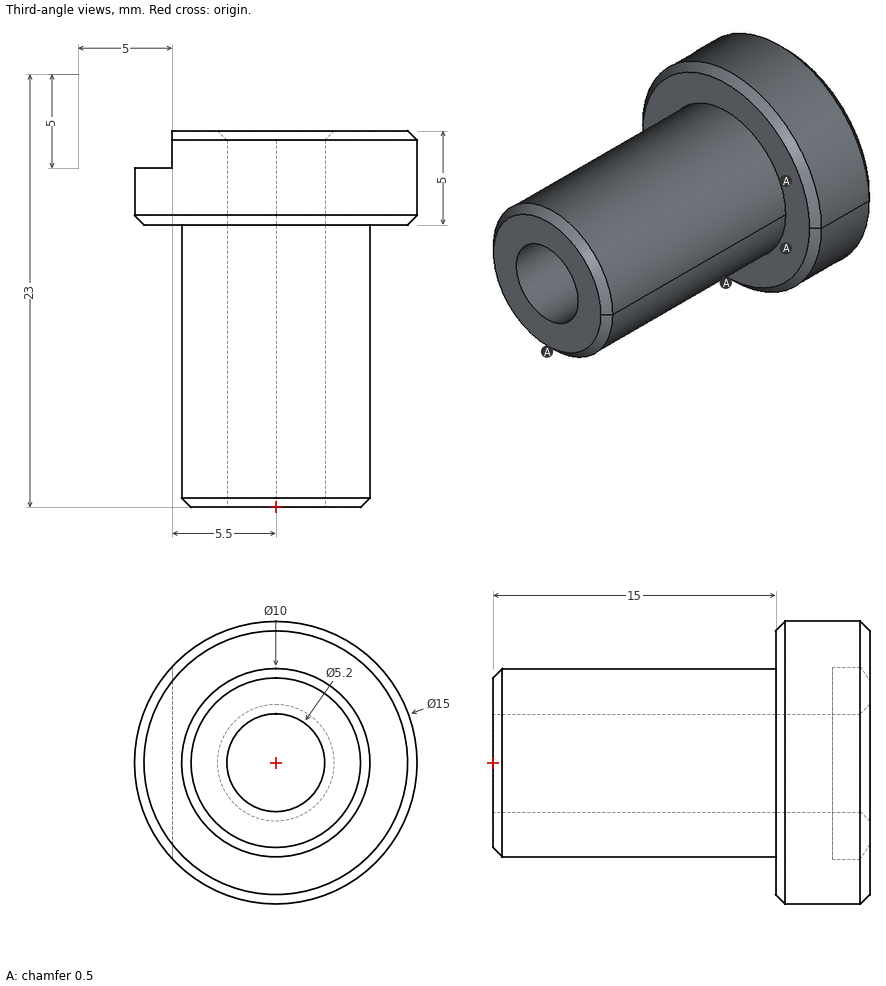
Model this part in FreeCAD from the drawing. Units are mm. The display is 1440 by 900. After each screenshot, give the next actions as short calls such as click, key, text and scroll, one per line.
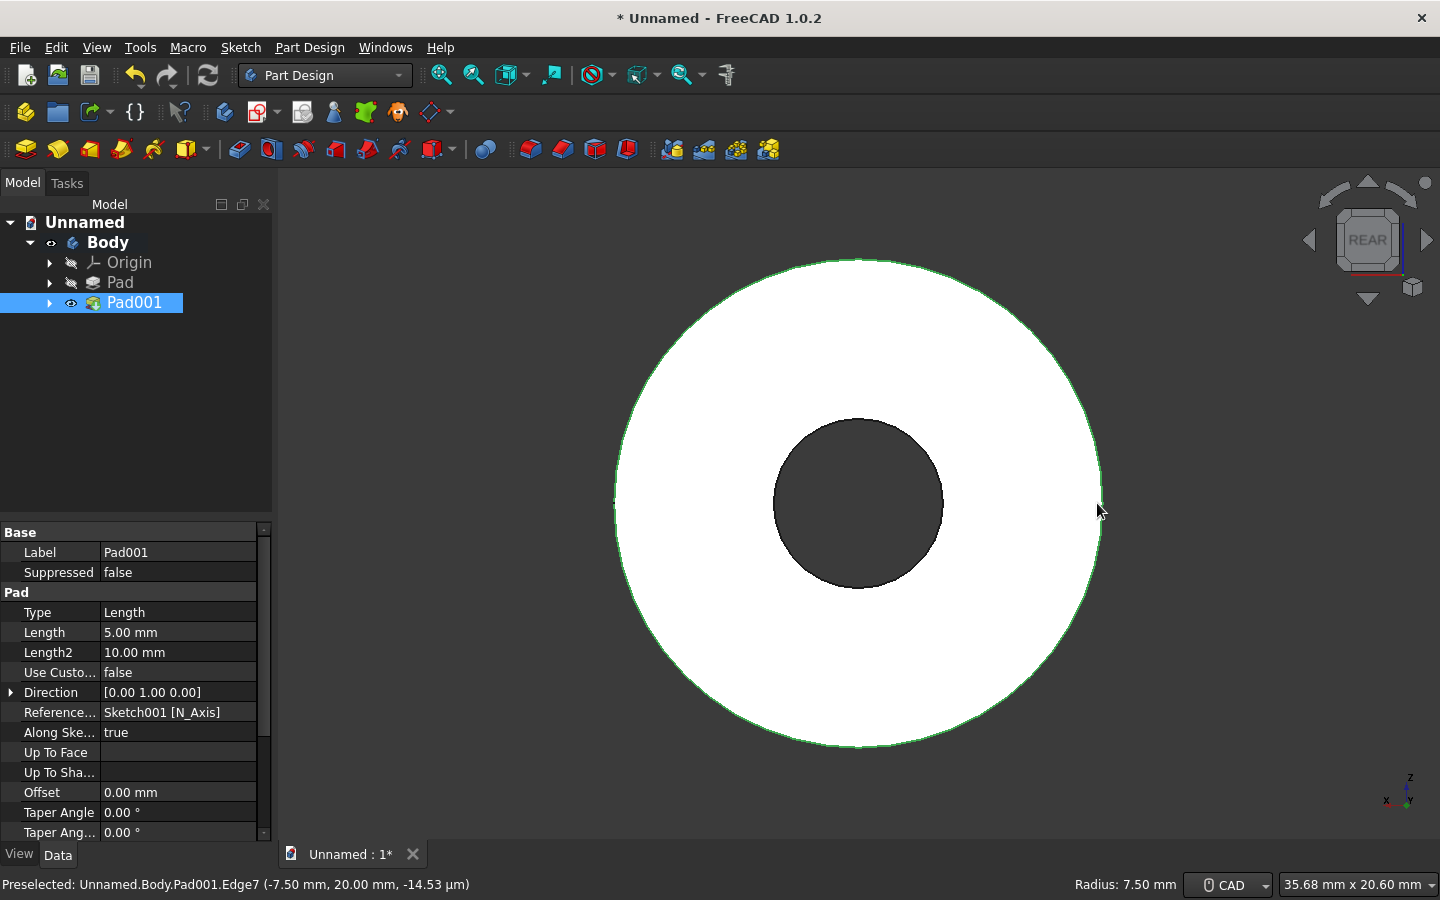
click(927, 453, ctrl)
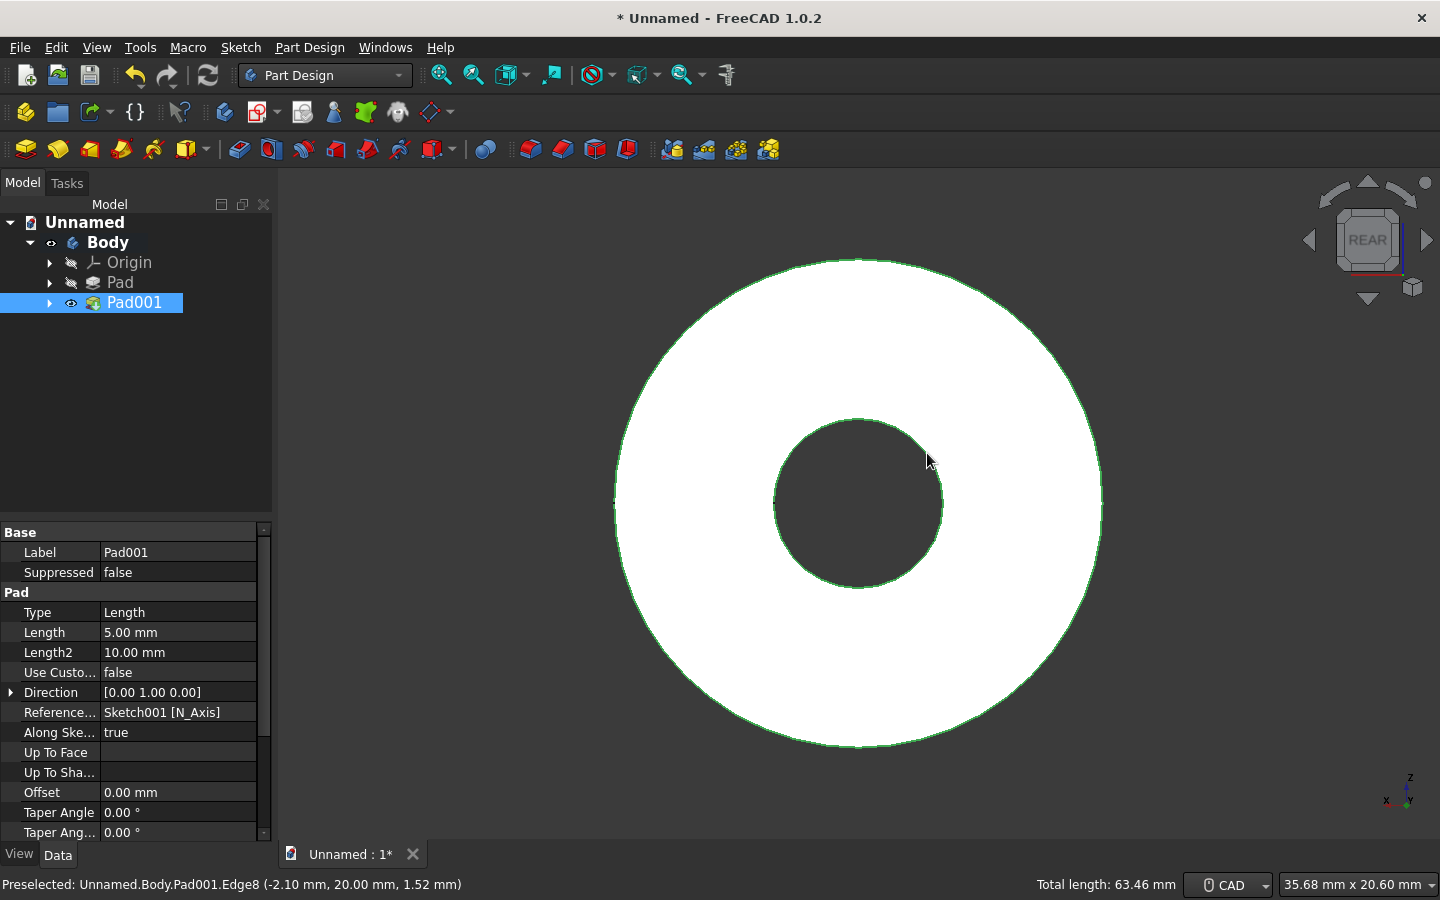
key(0)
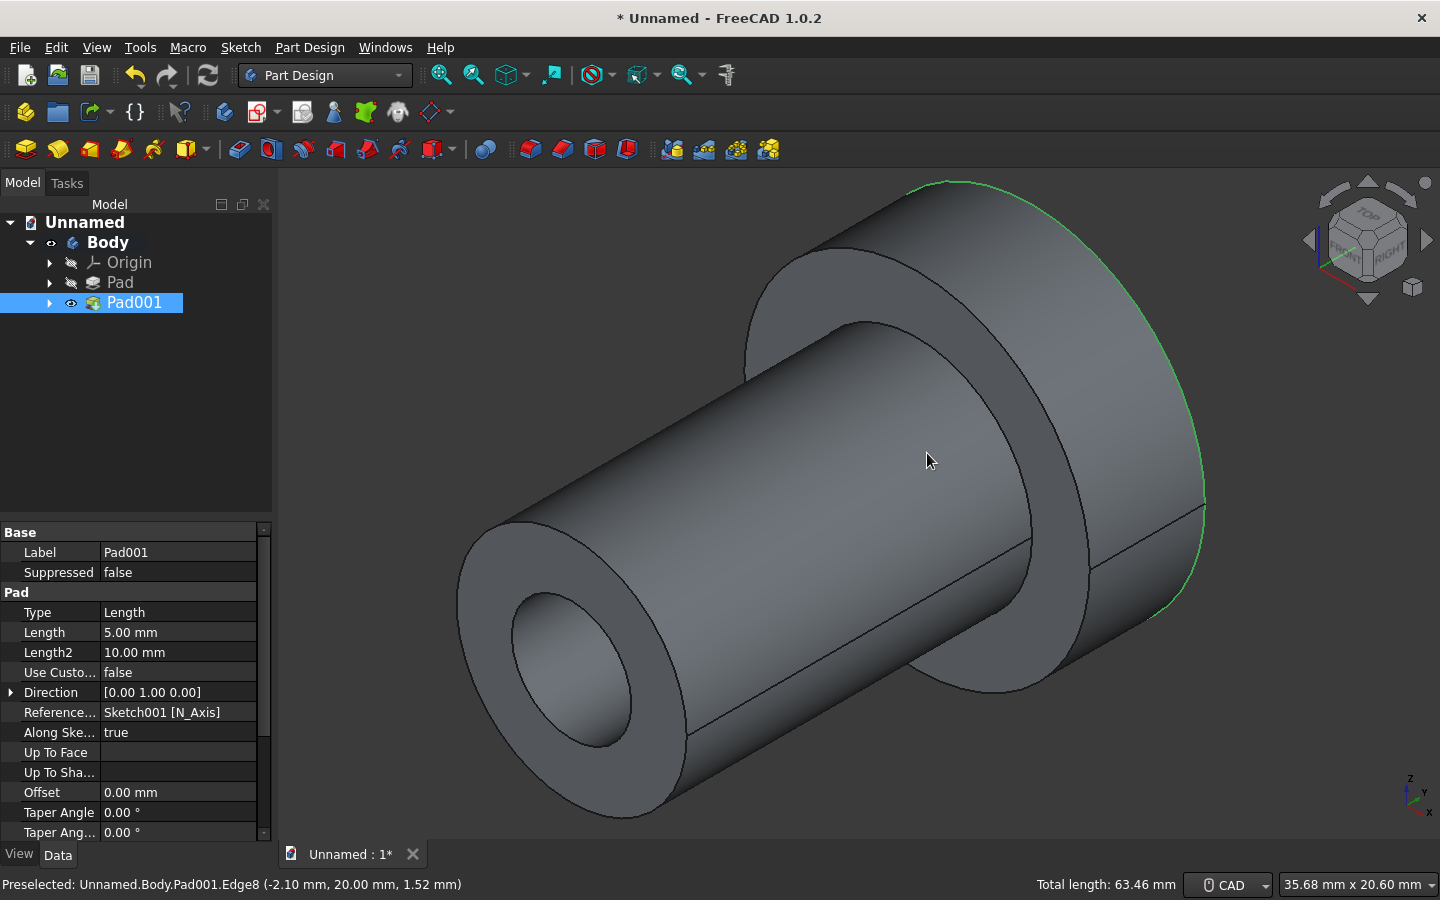
click(442, 76)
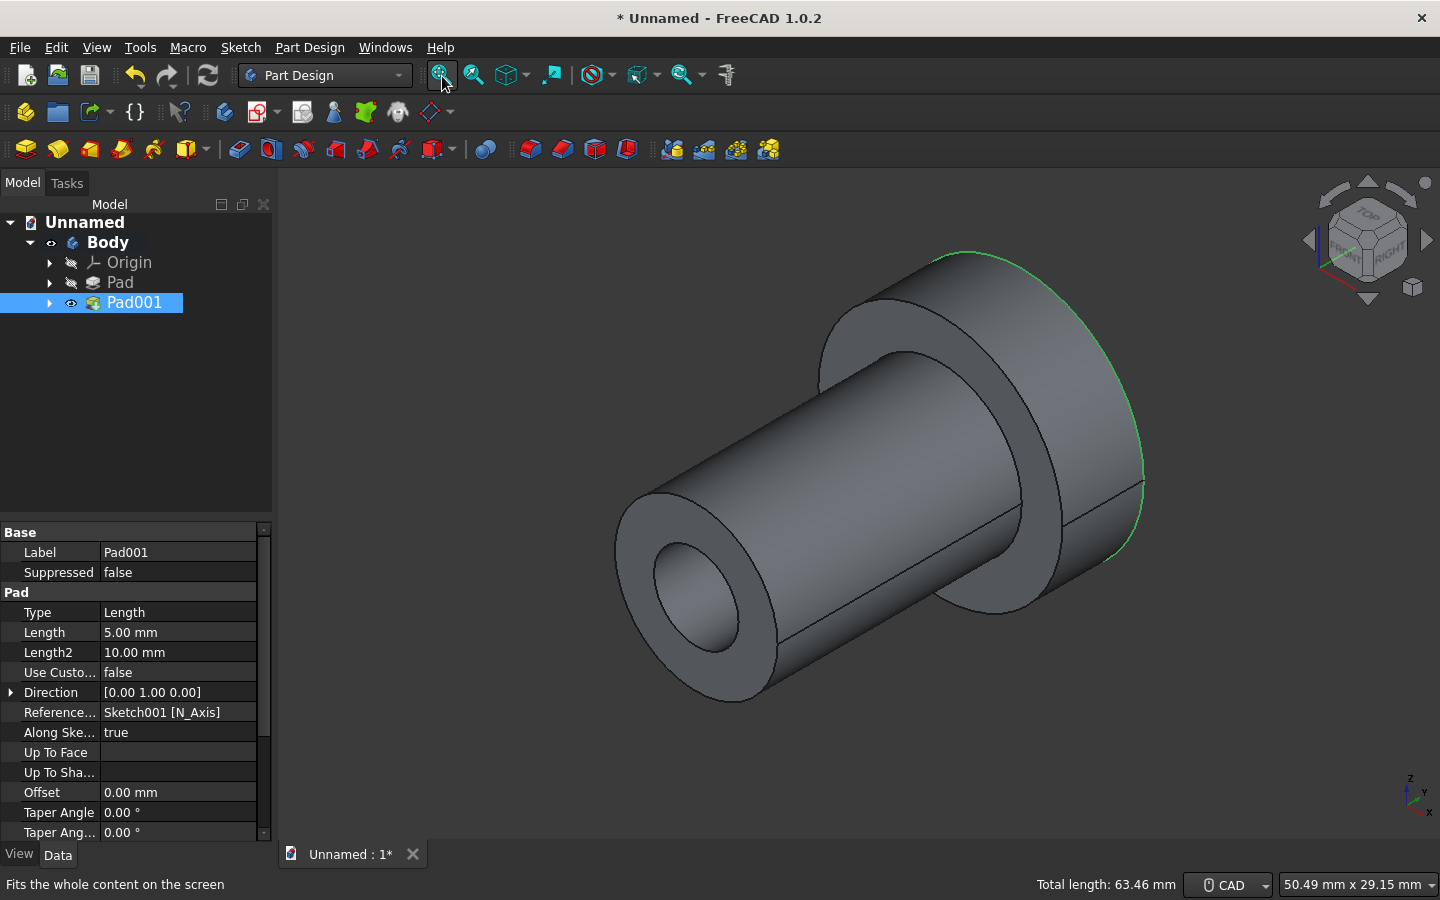
click(903, 300, ctrl)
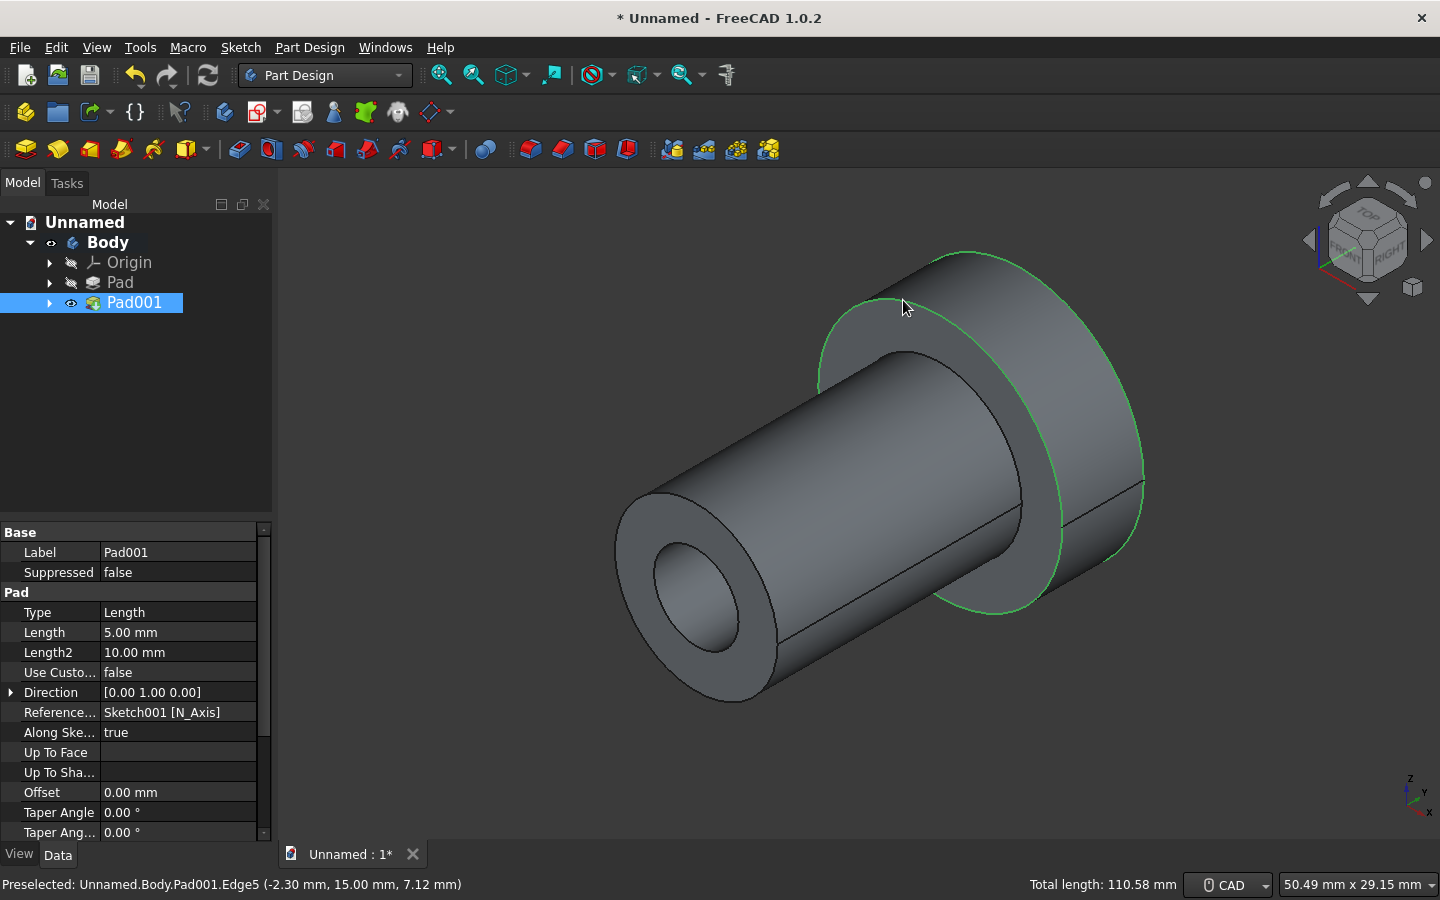
click(671, 493, ctrl)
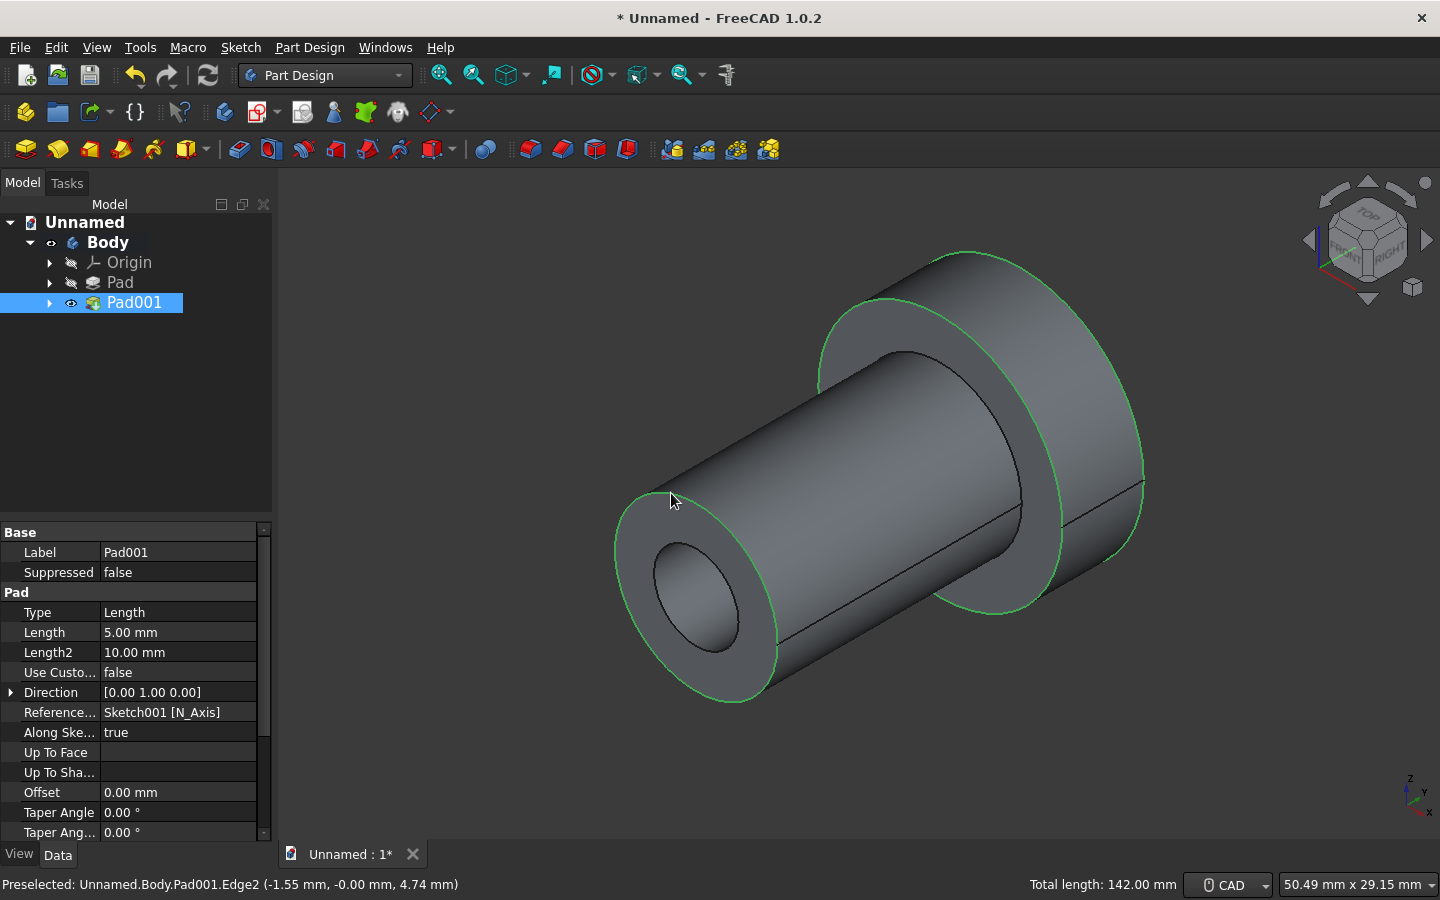
click(564, 150)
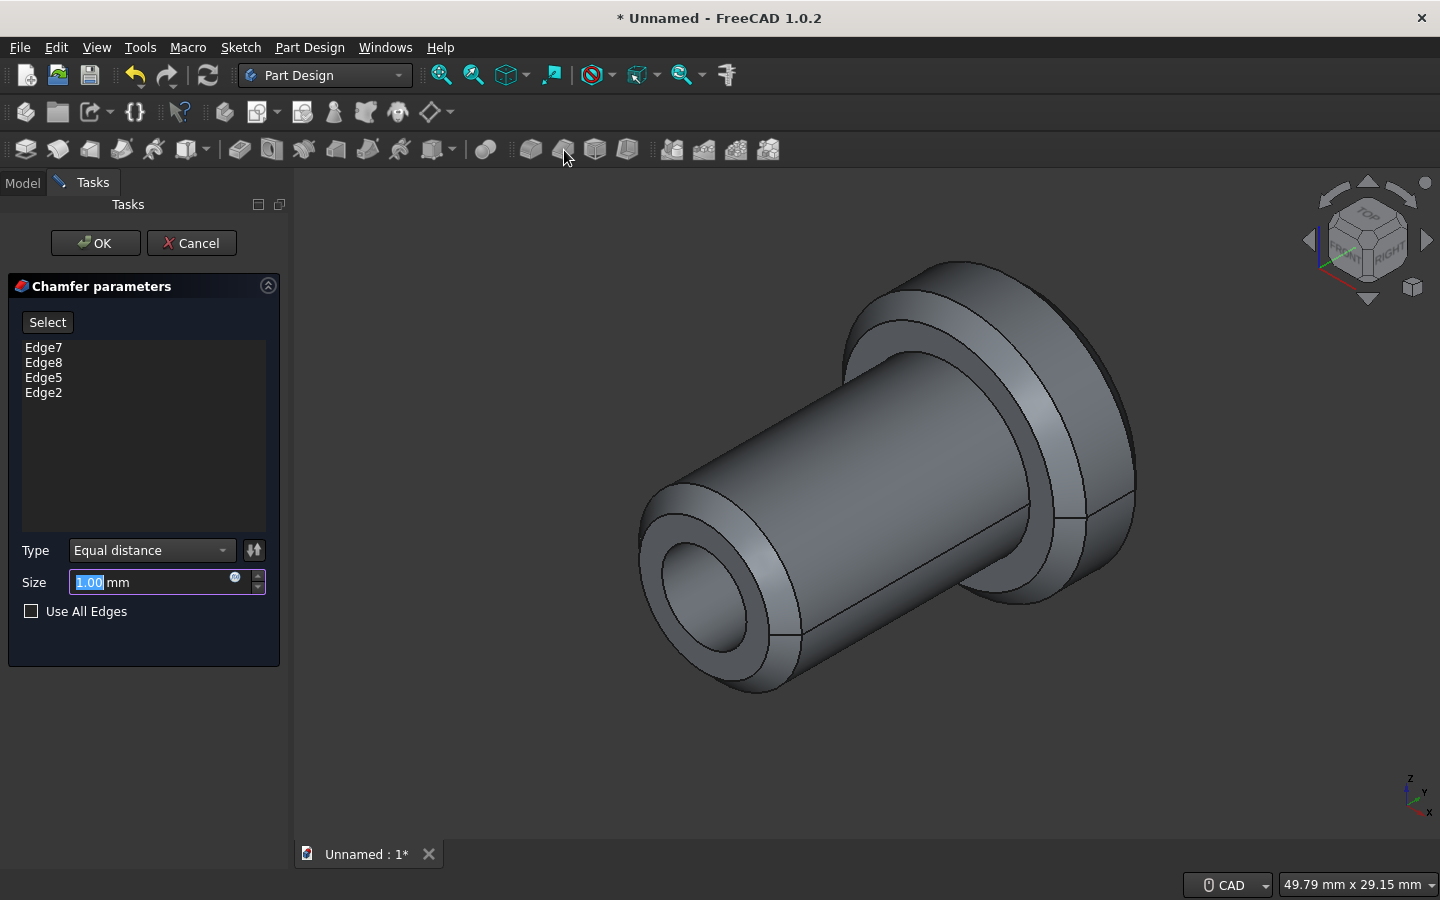
text(0.5)
key(Tab)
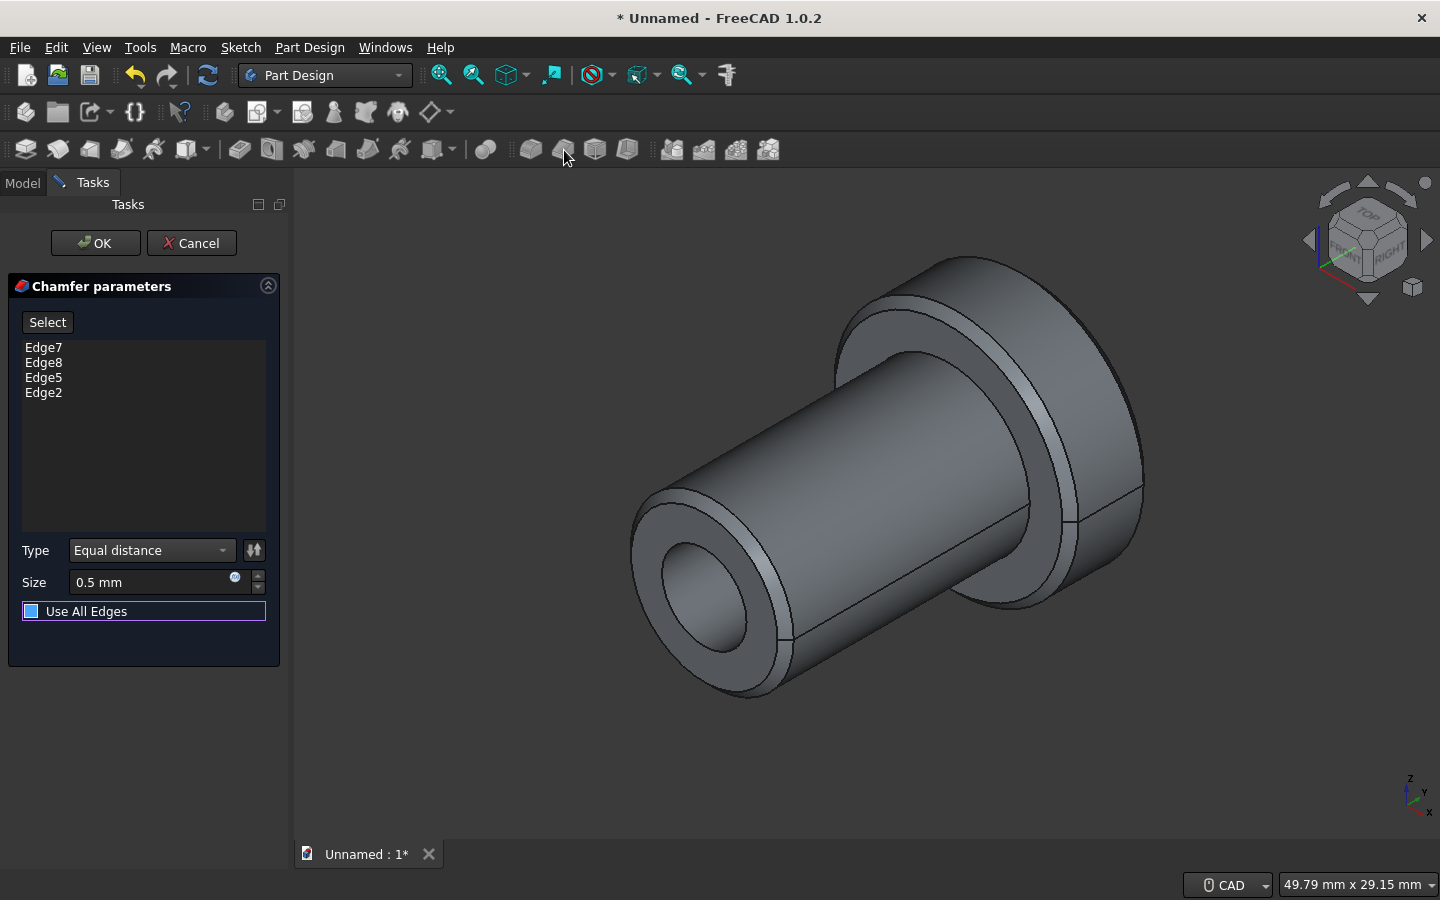
click(96, 243)